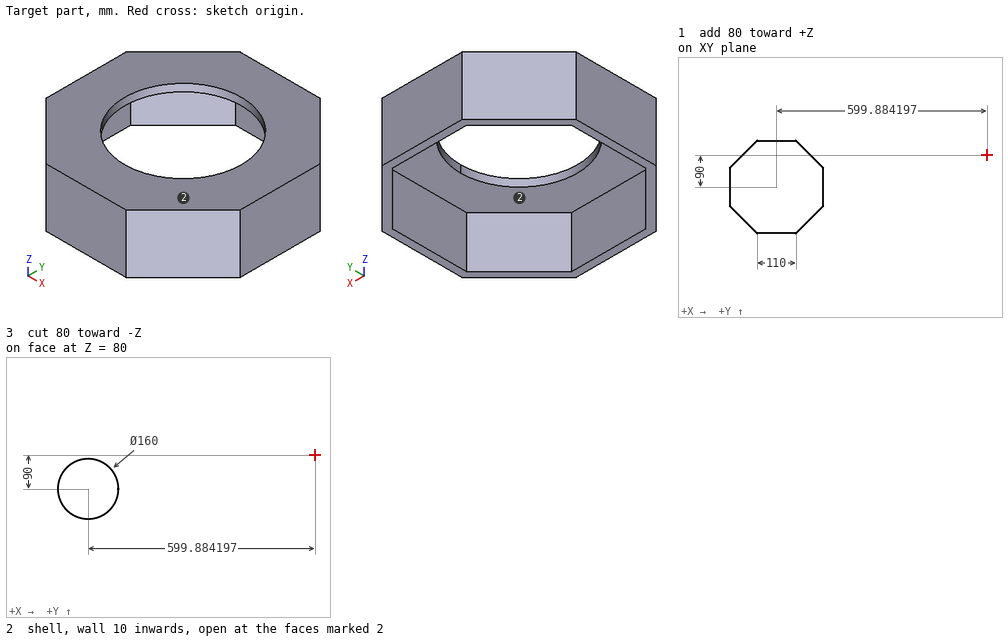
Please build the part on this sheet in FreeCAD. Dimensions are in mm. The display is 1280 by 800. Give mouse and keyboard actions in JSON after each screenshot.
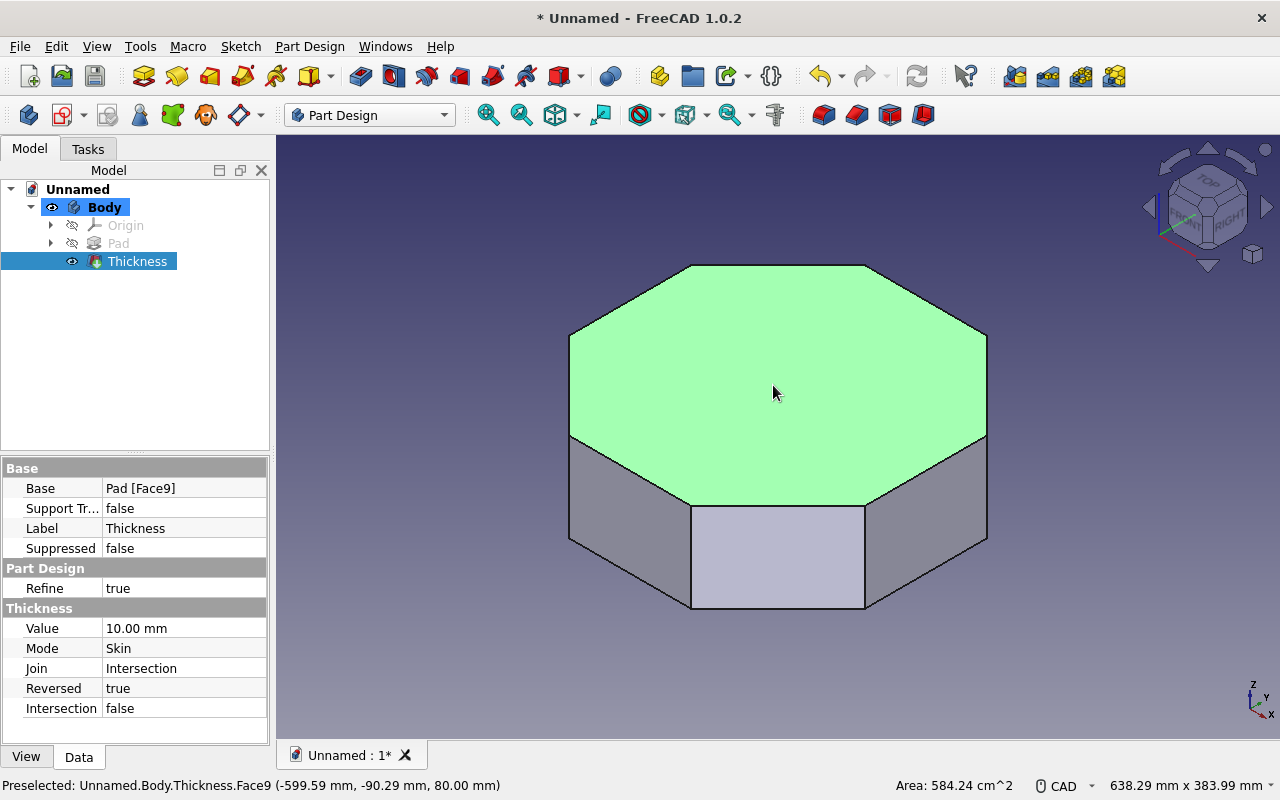
{"action": "left_click", "coordinate": [62, 116]}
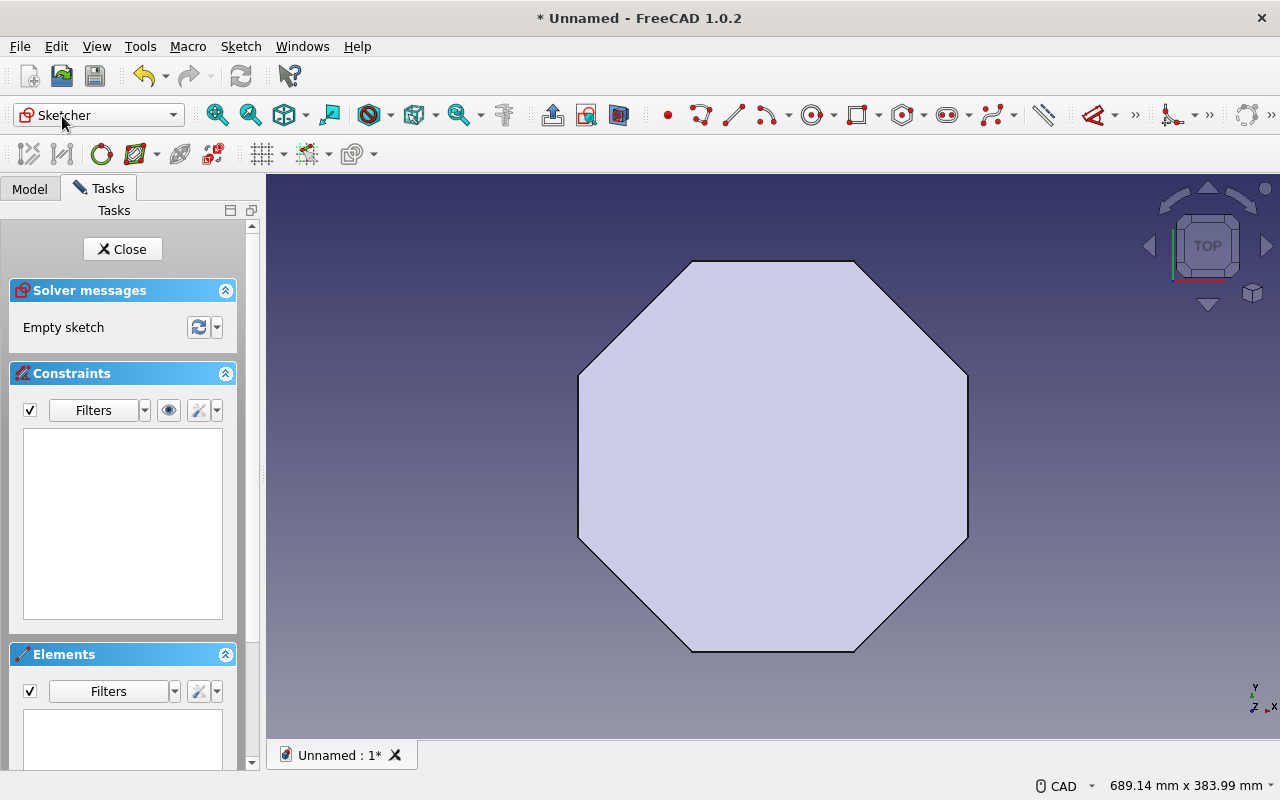
{"action": "scroll", "coordinate": [912, 457], "scroll_direction": "up", "scroll_amount": 2}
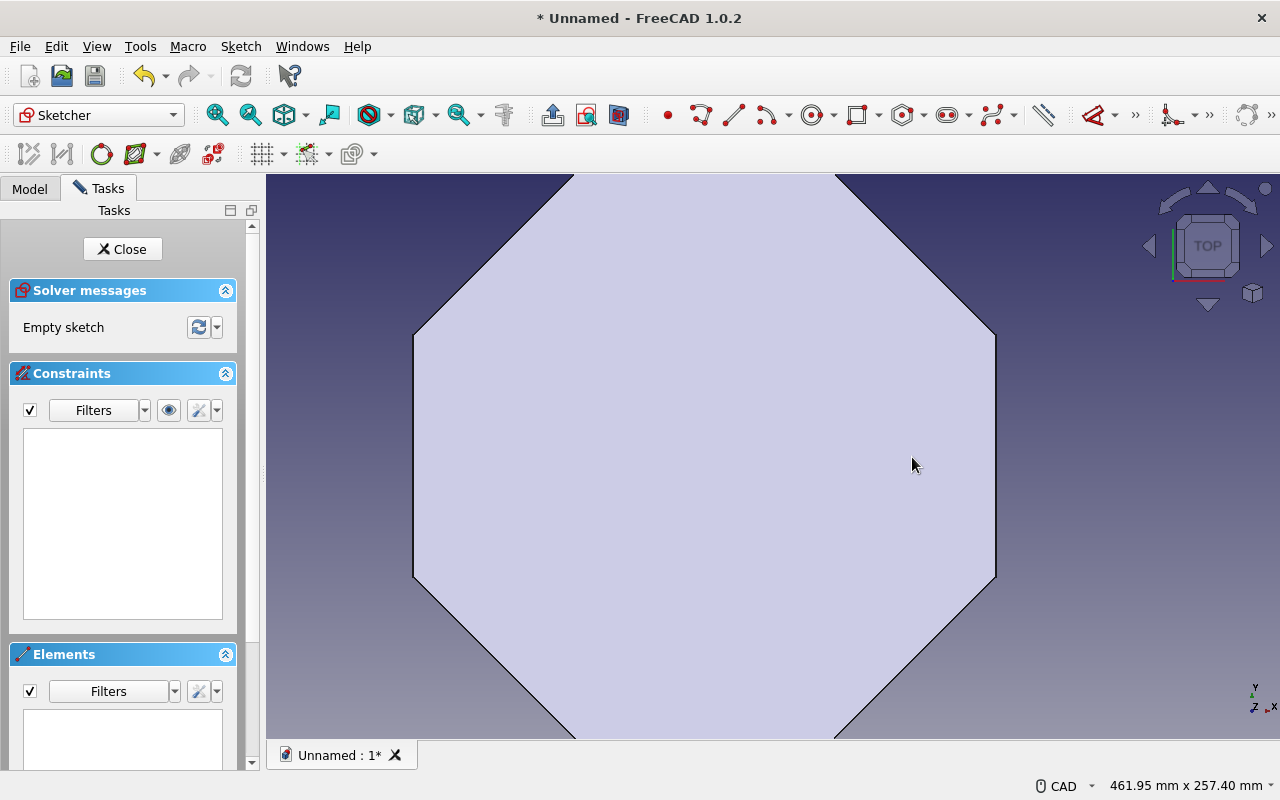
{"action": "left_click", "coordinate": [812, 116]}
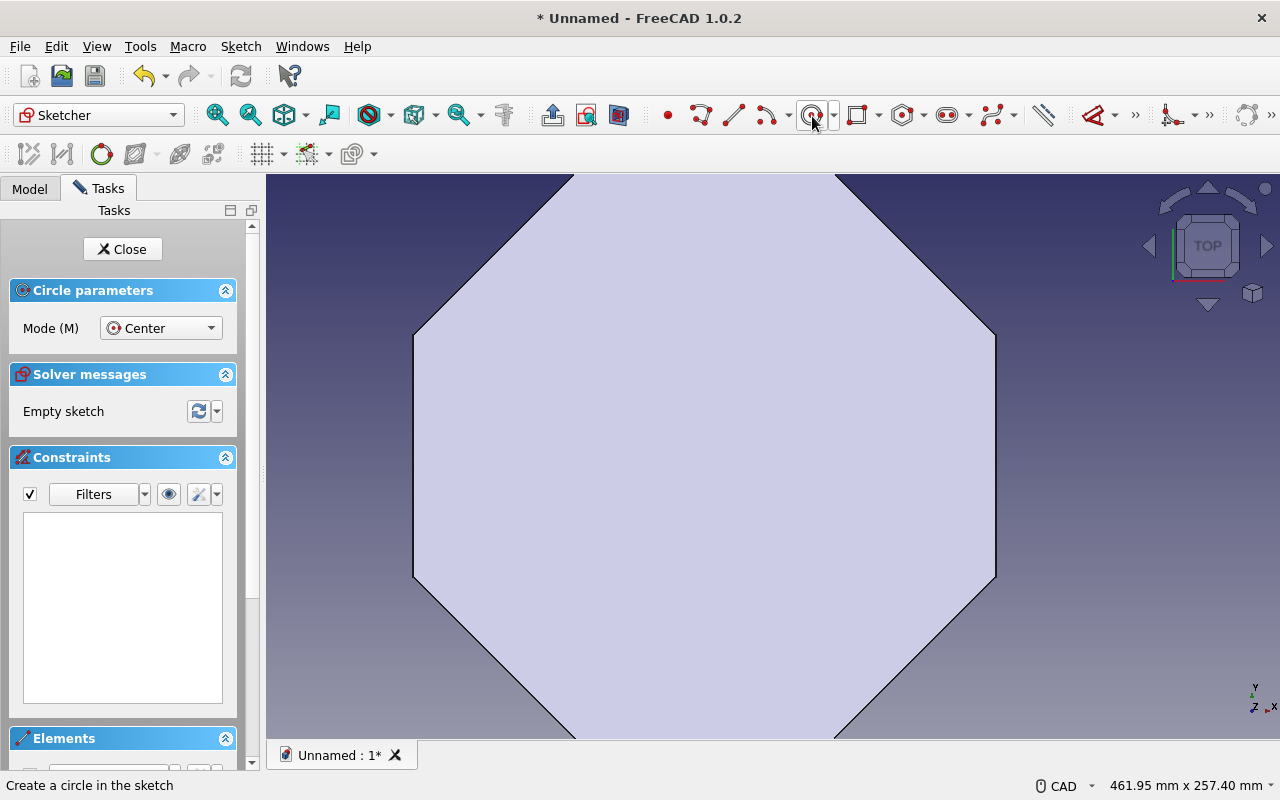
{"action": "left_click", "coordinate": [704, 456]}
{"action": "mouse_move", "coordinate": [828, 332]}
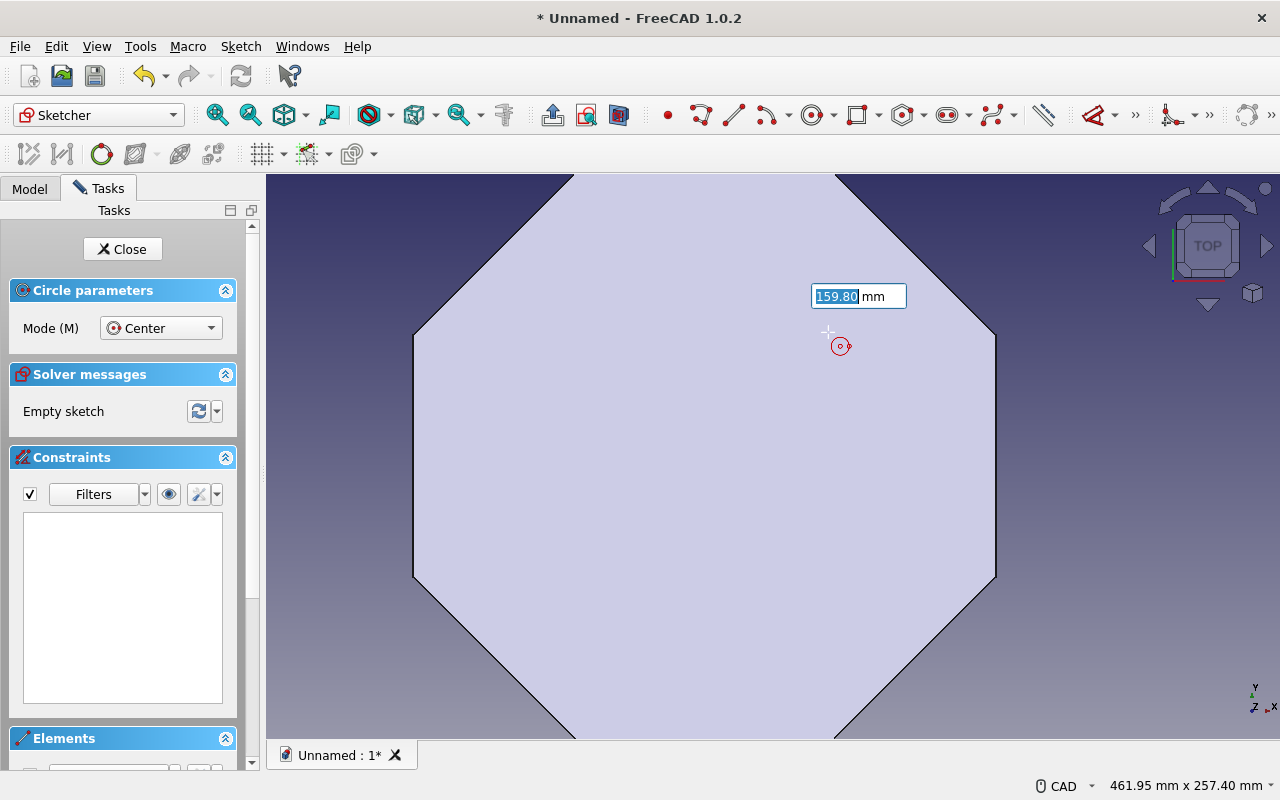
{"action": "type", "text": "160"}
{"action": "key", "text": "Return"}
{"action": "key", "text": "Escape"}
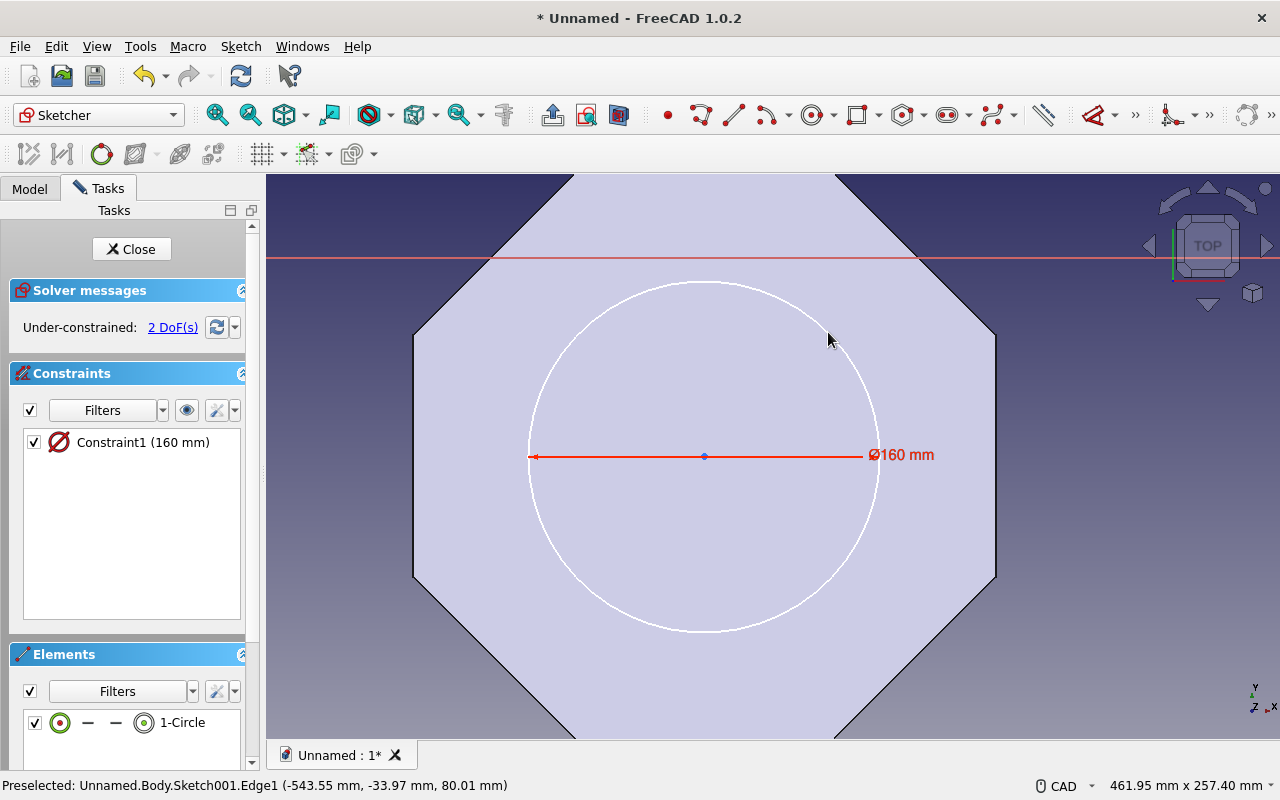
{"action": "left_click", "coordinate": [704, 457]}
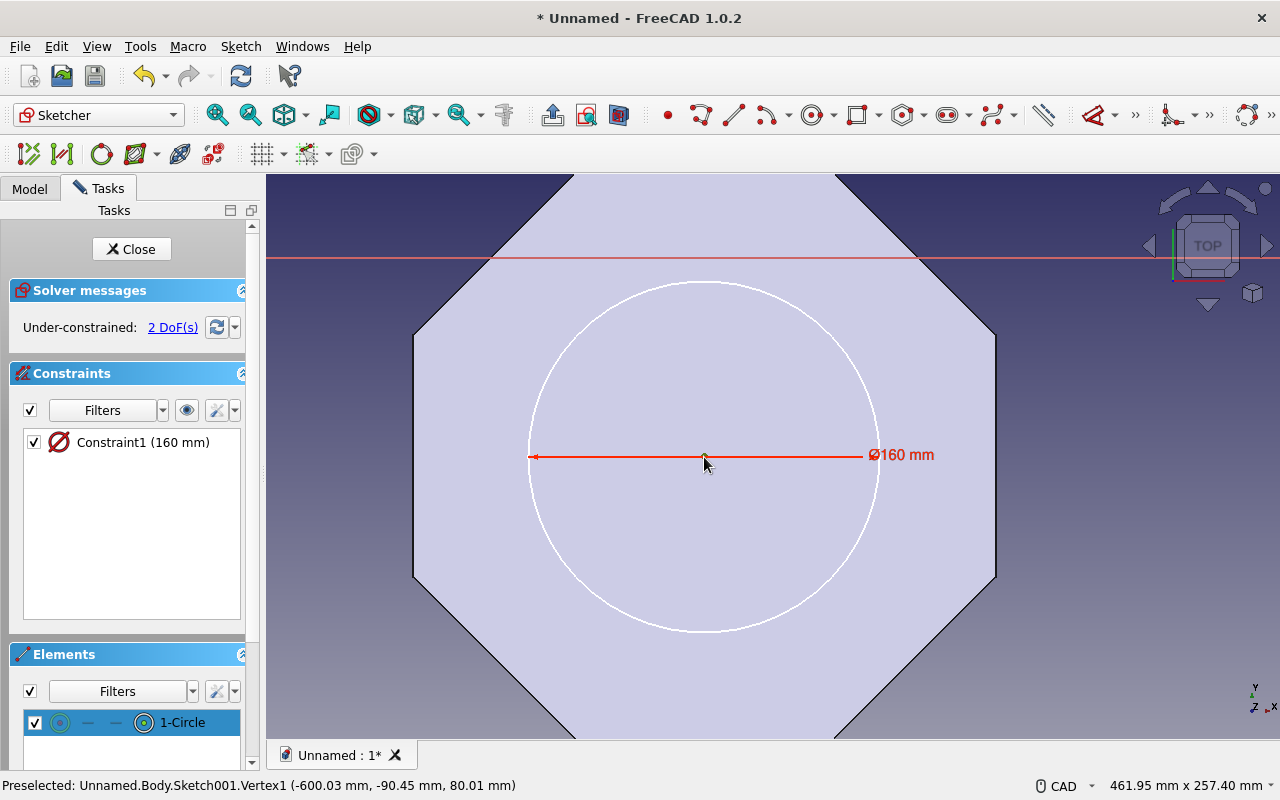
{"action": "key", "text": "i"}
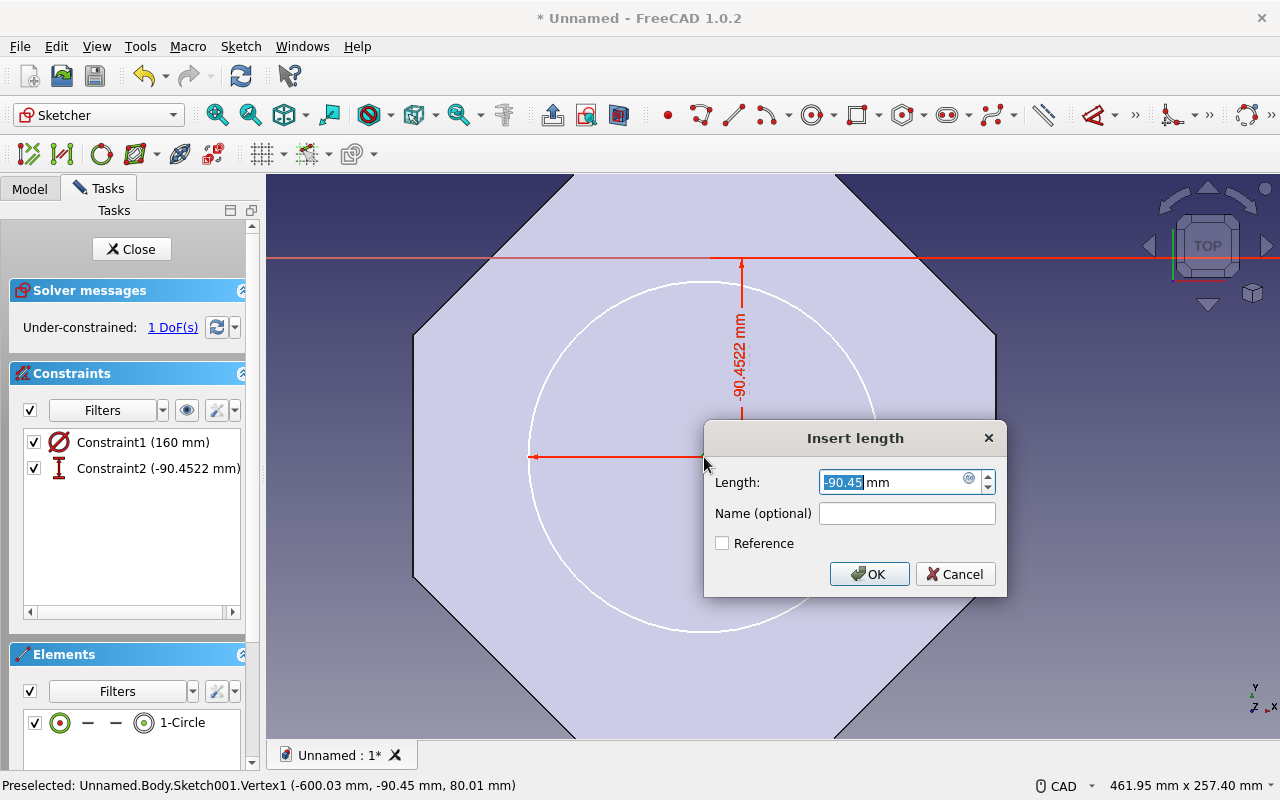
{"action": "type", "text": "-90"}
{"action": "key", "text": "Return"}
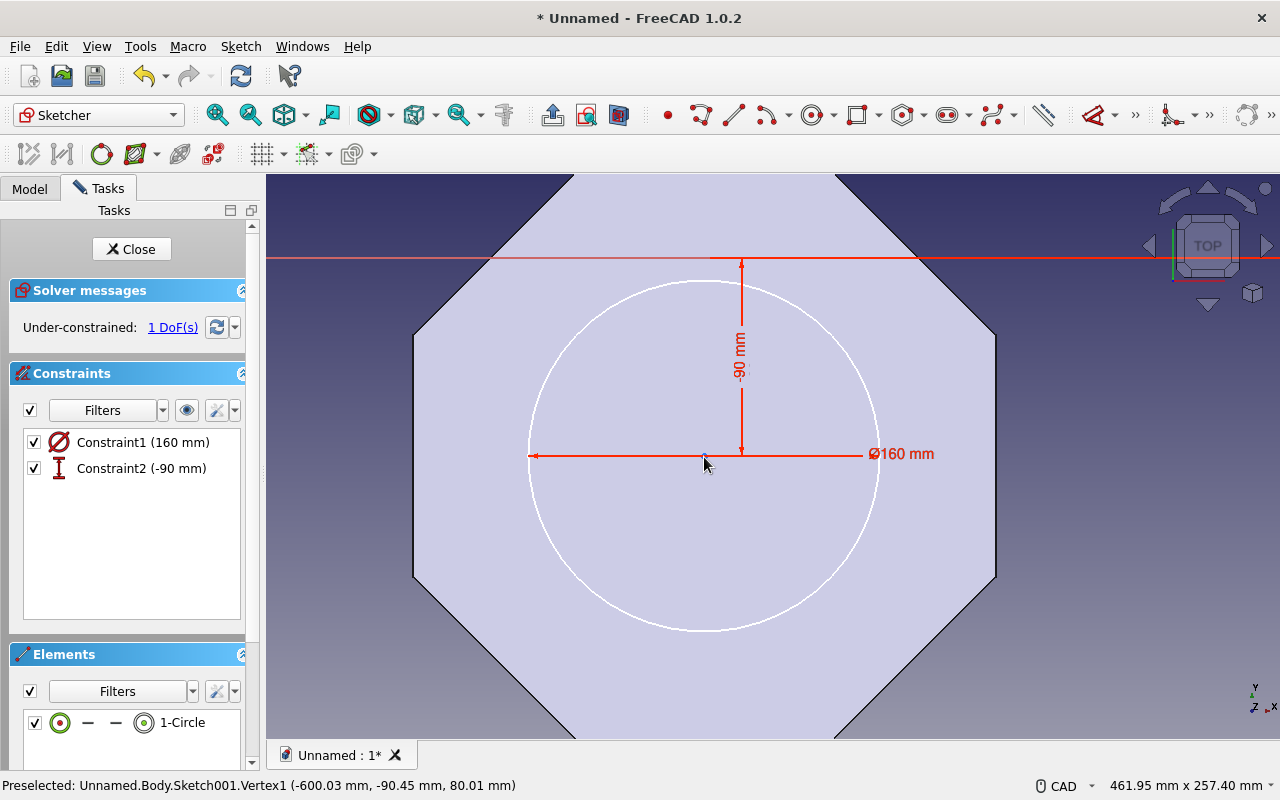
{"action": "left_click", "coordinate": [704, 456]}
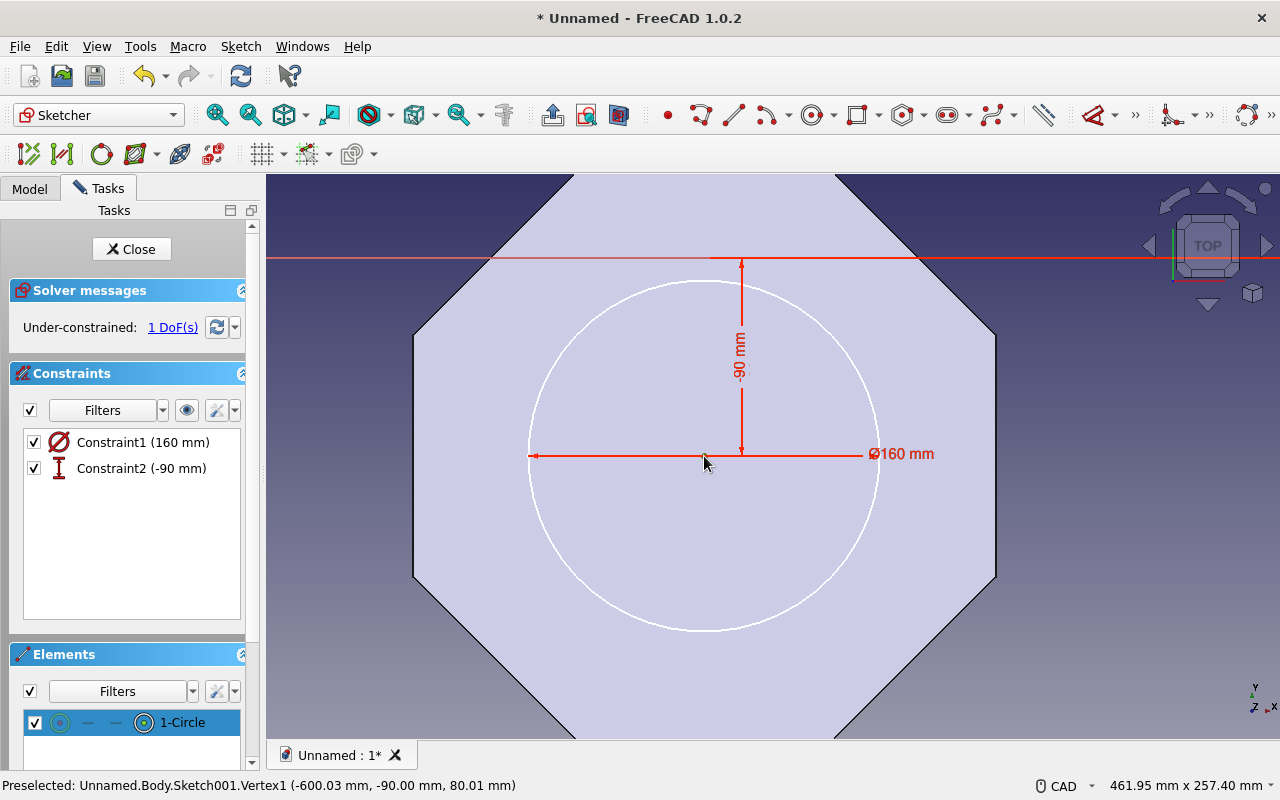
{"action": "key", "text": "l"}